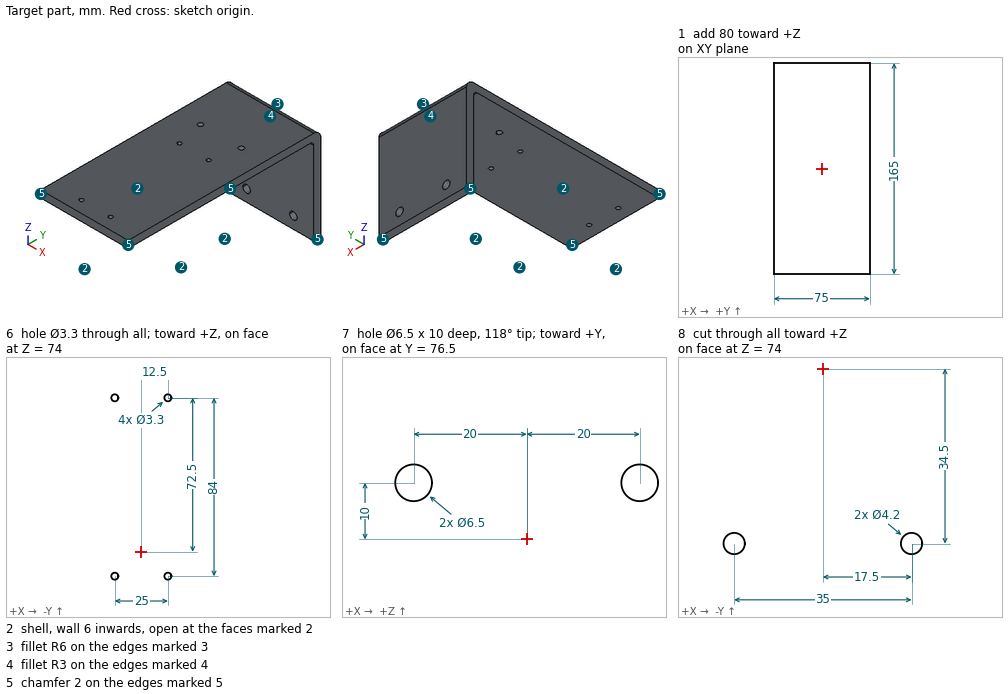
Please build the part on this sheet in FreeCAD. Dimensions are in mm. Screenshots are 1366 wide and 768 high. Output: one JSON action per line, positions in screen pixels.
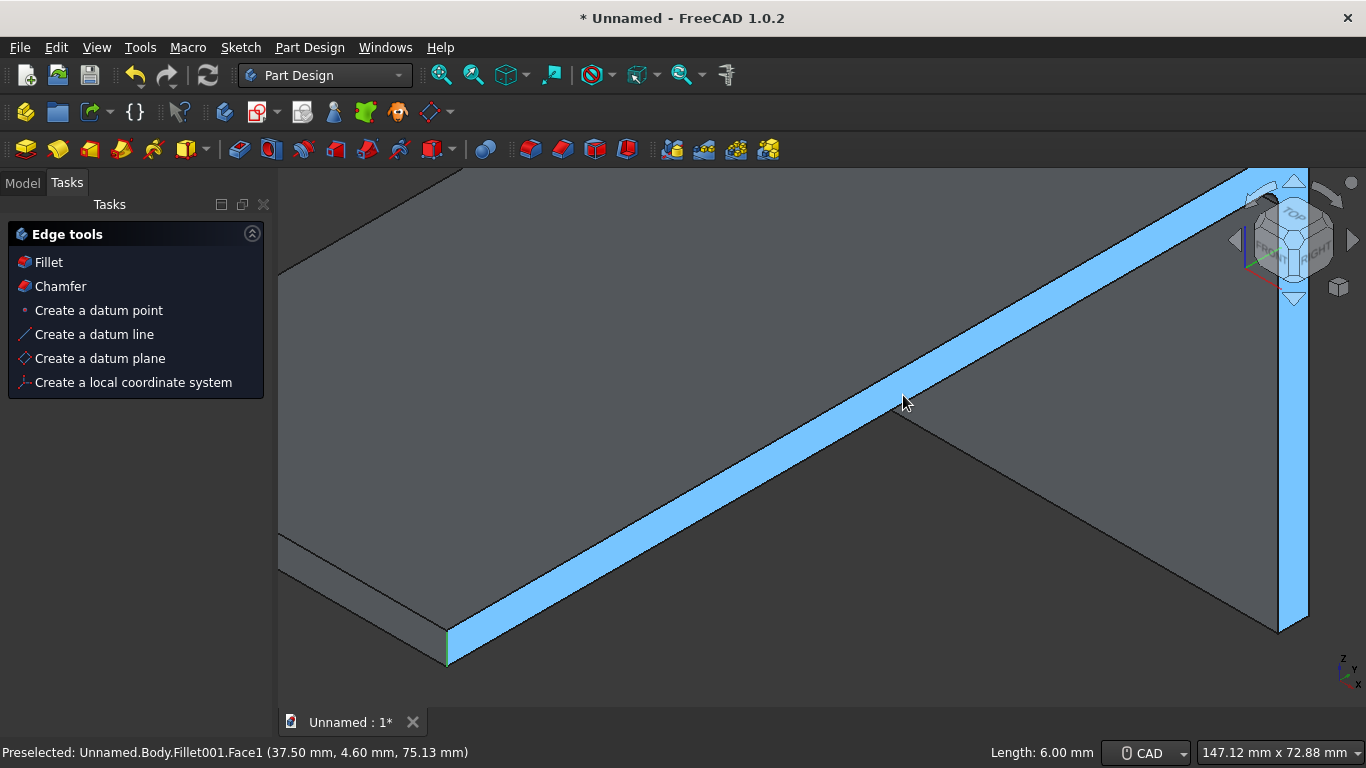
{"action": "left_click", "coordinate": [442, 76]}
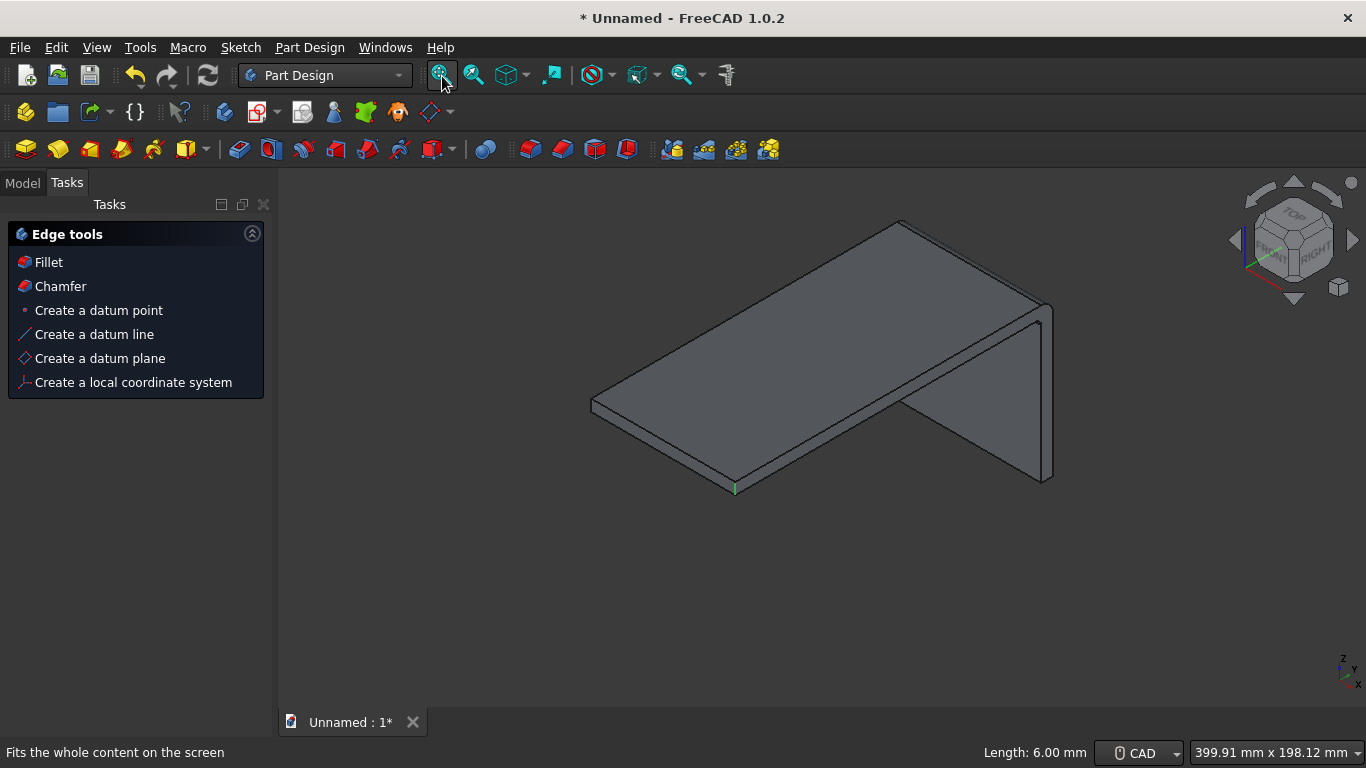
{"action": "key", "text": "1"}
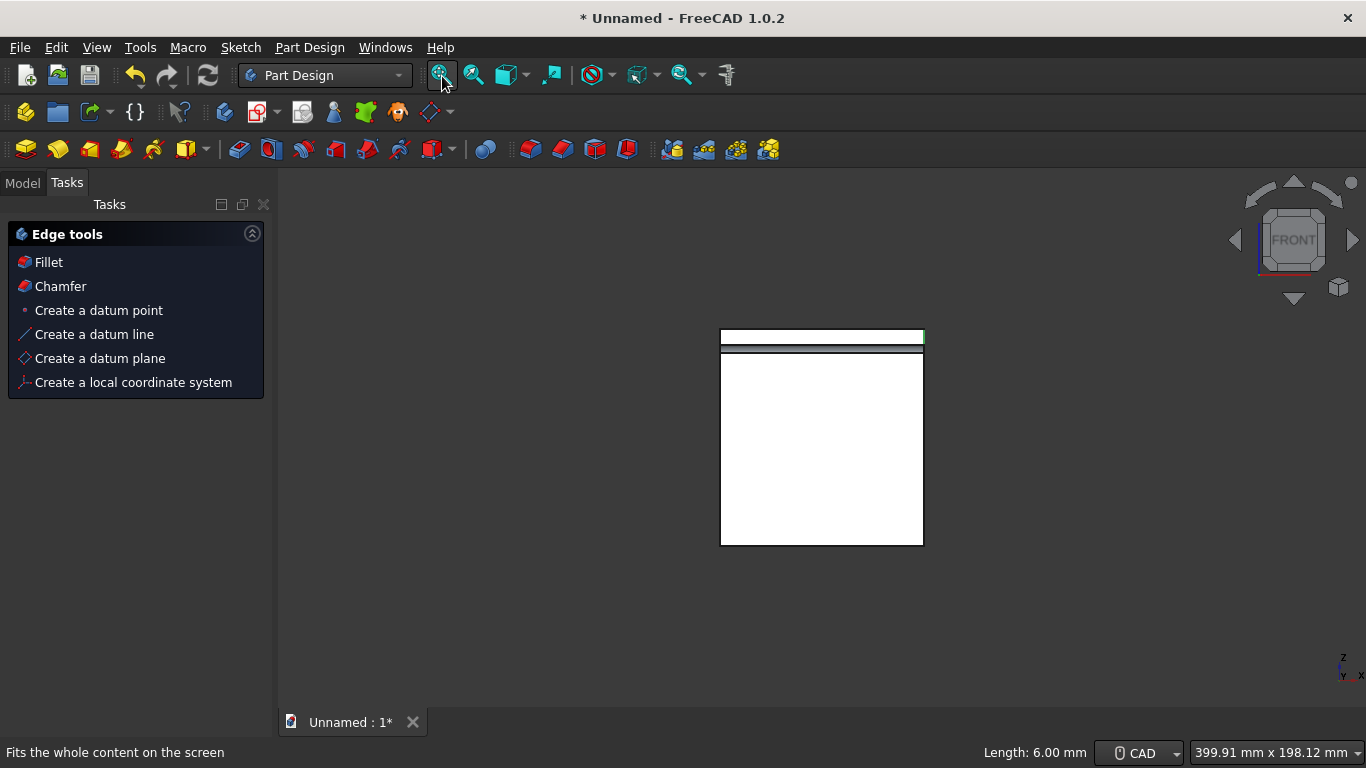
{"action": "left_click", "coordinate": [442, 76]}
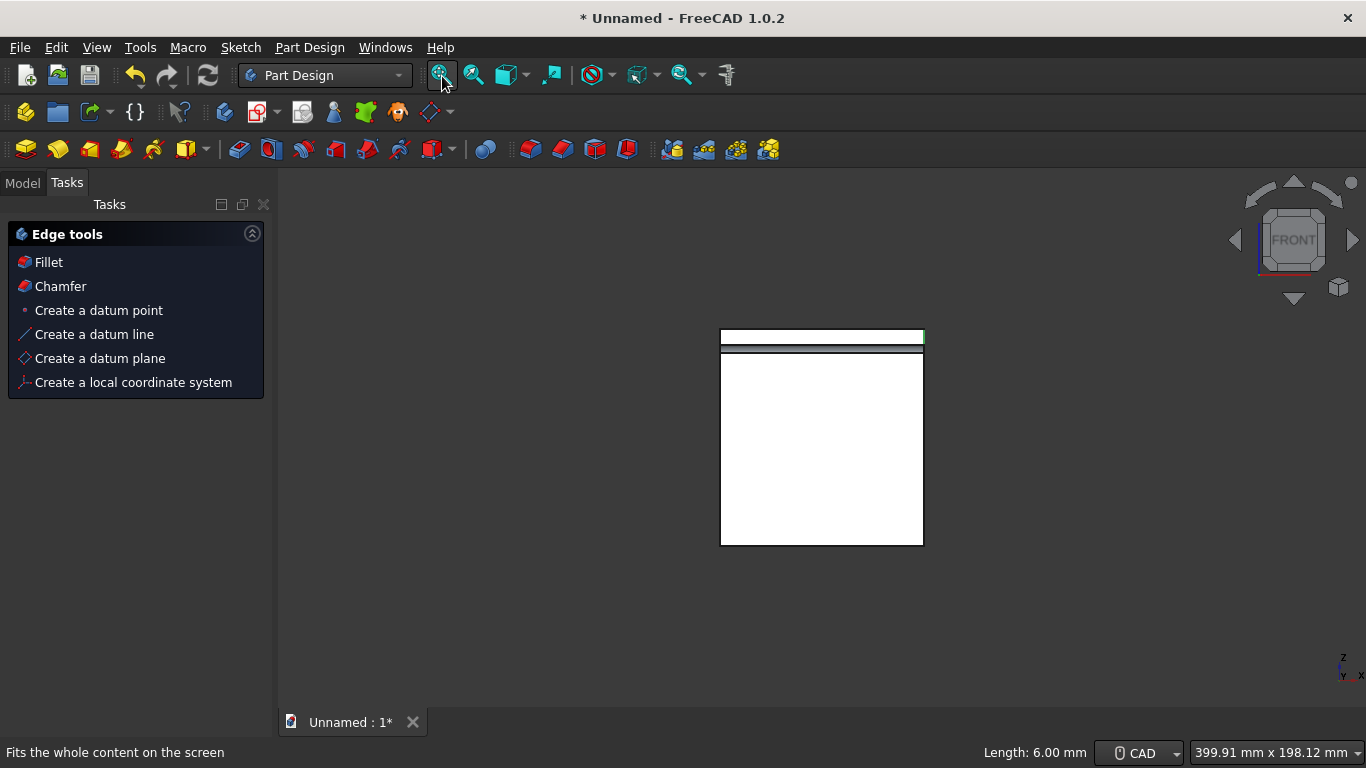
{"action": "left_click", "coordinate": [720, 336], "text": "ctrl"}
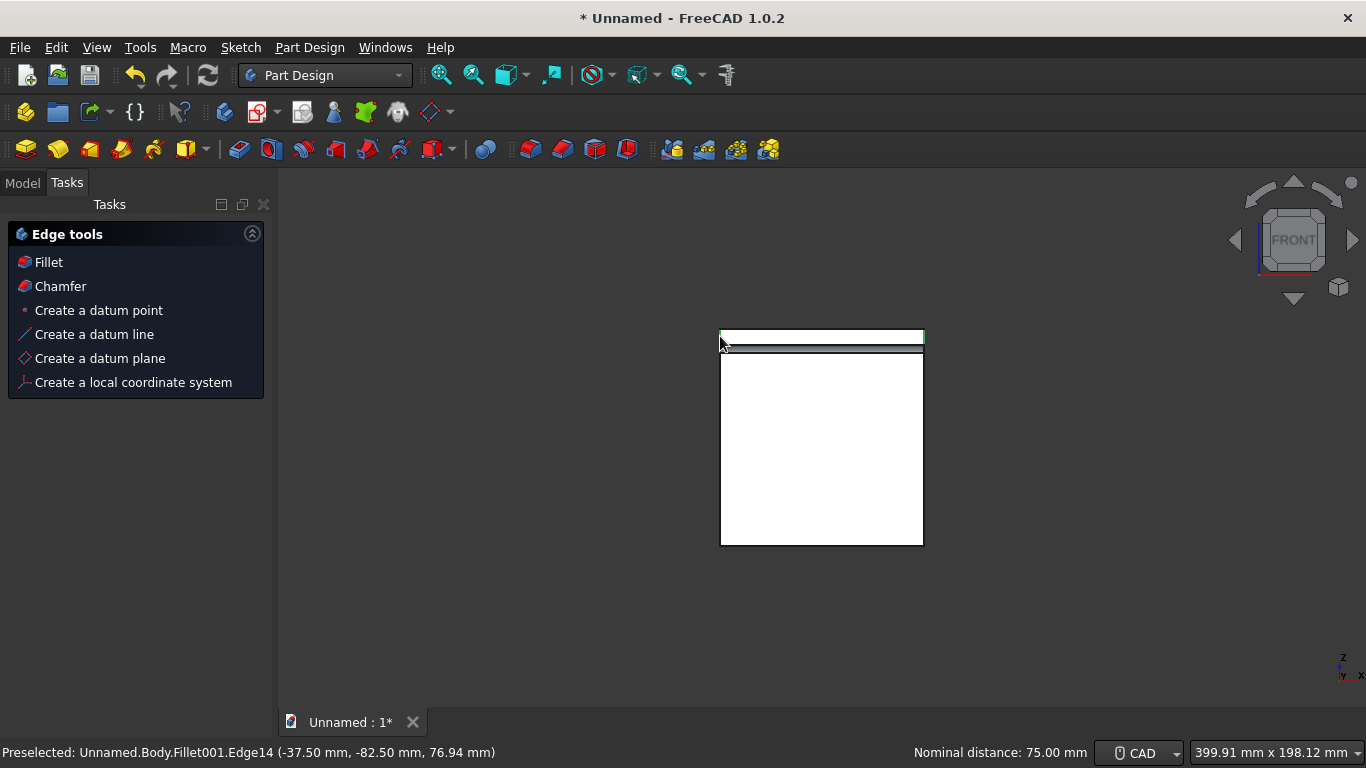
{"action": "scroll", "coordinate": [720, 545], "scroll_direction": "up", "scroll_amount": 5}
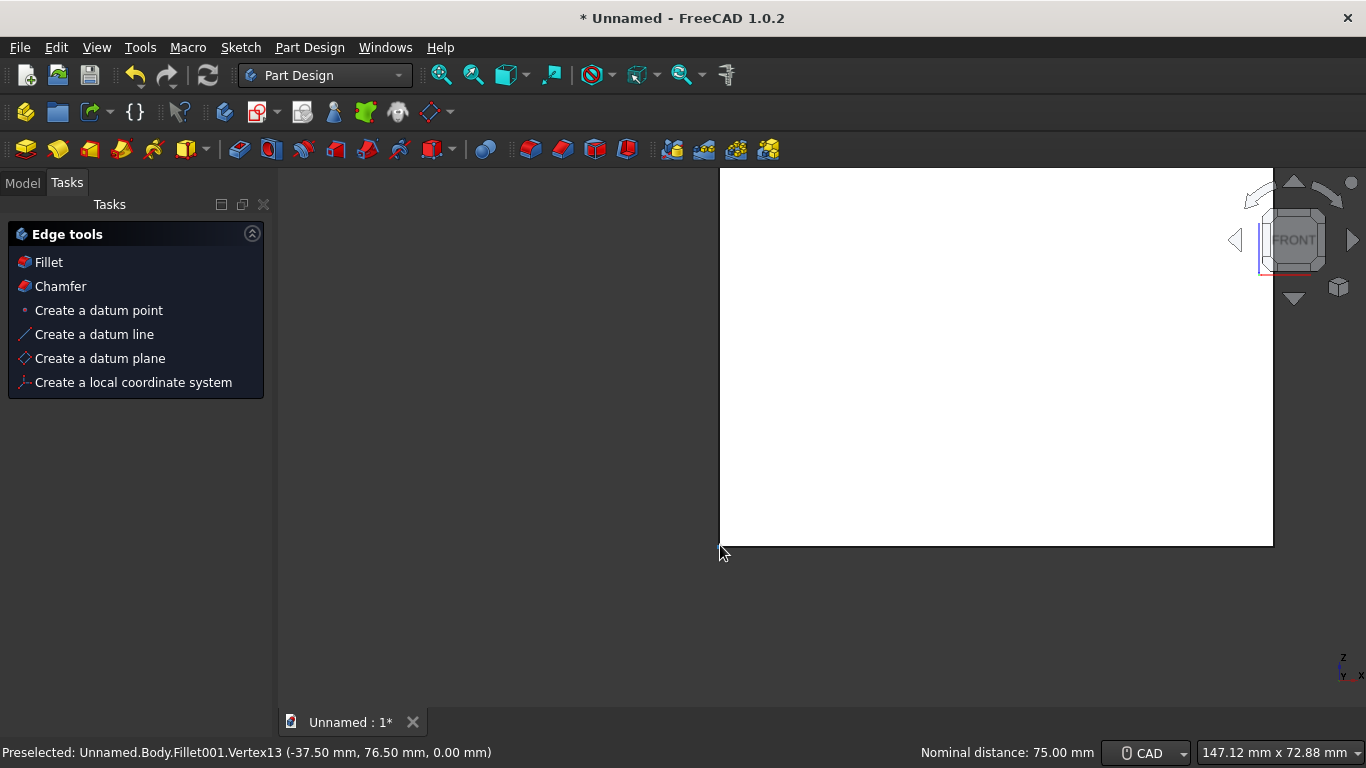
{"action": "left_click", "coordinate": [442, 76]}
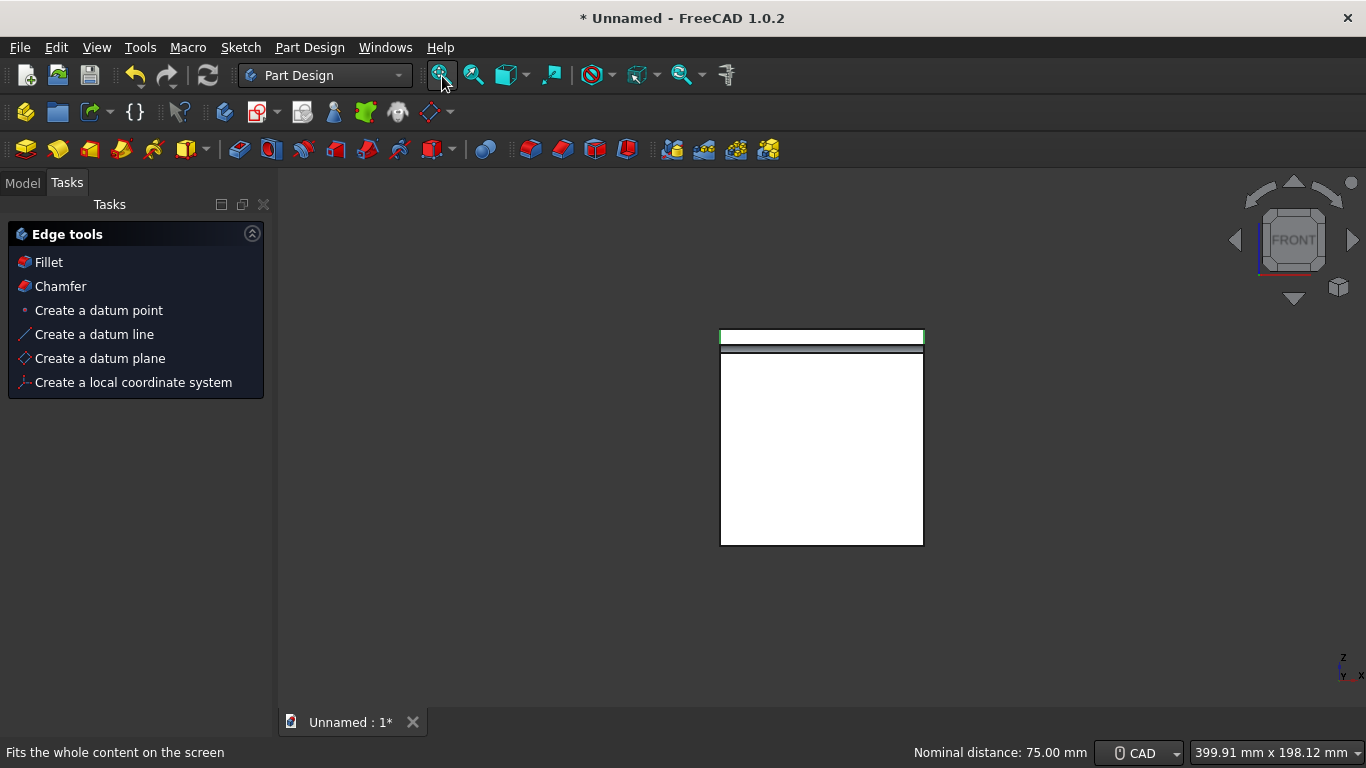
{"action": "key", "text": "3"}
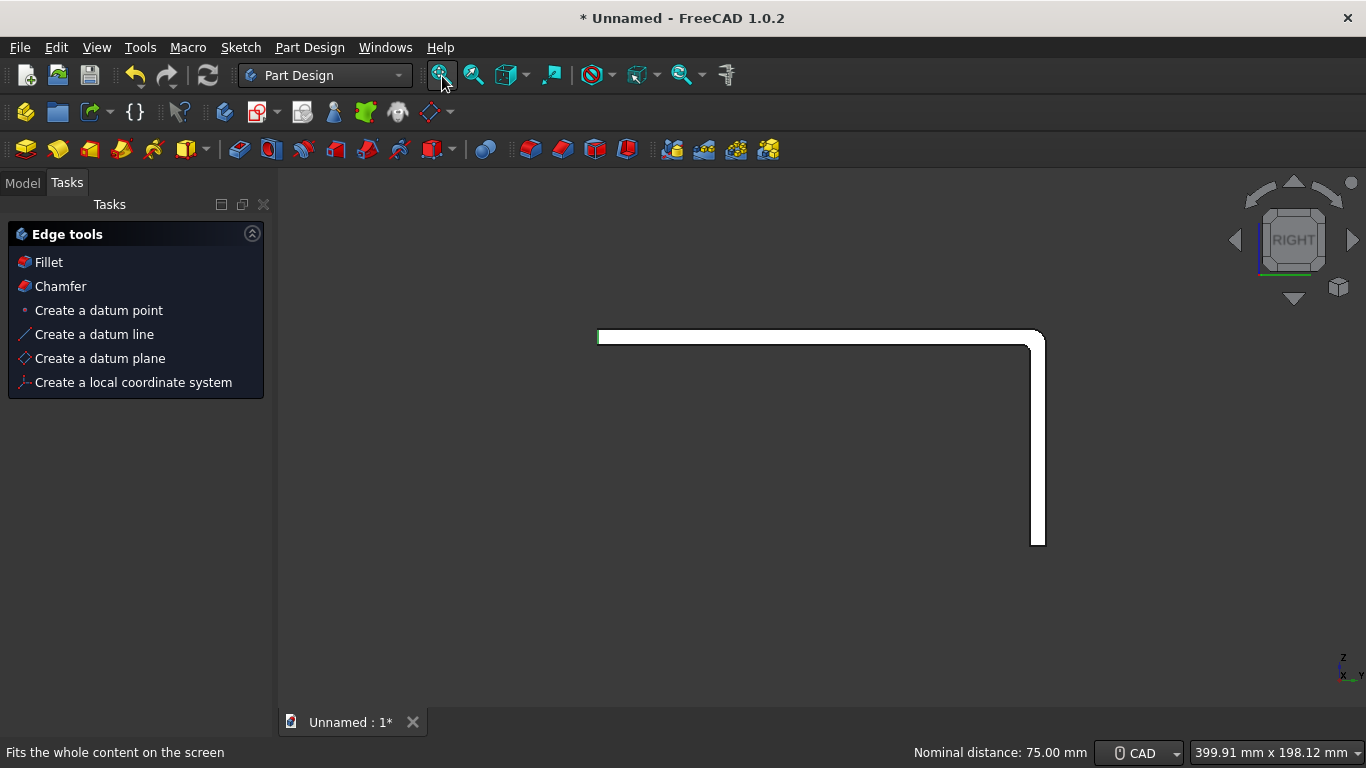
{"action": "left_click", "coordinate": [442, 76]}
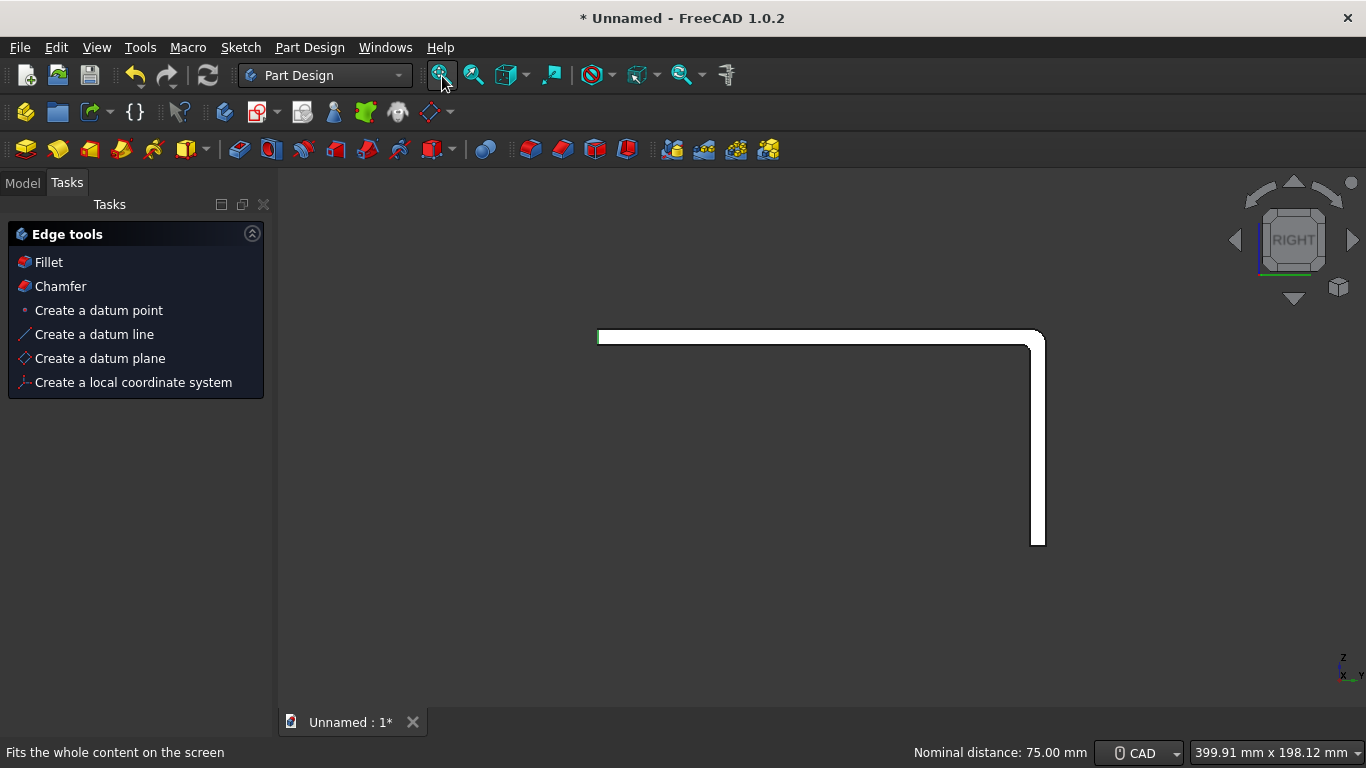
{"action": "left_click", "coordinate": [1038, 545], "text": "ctrl"}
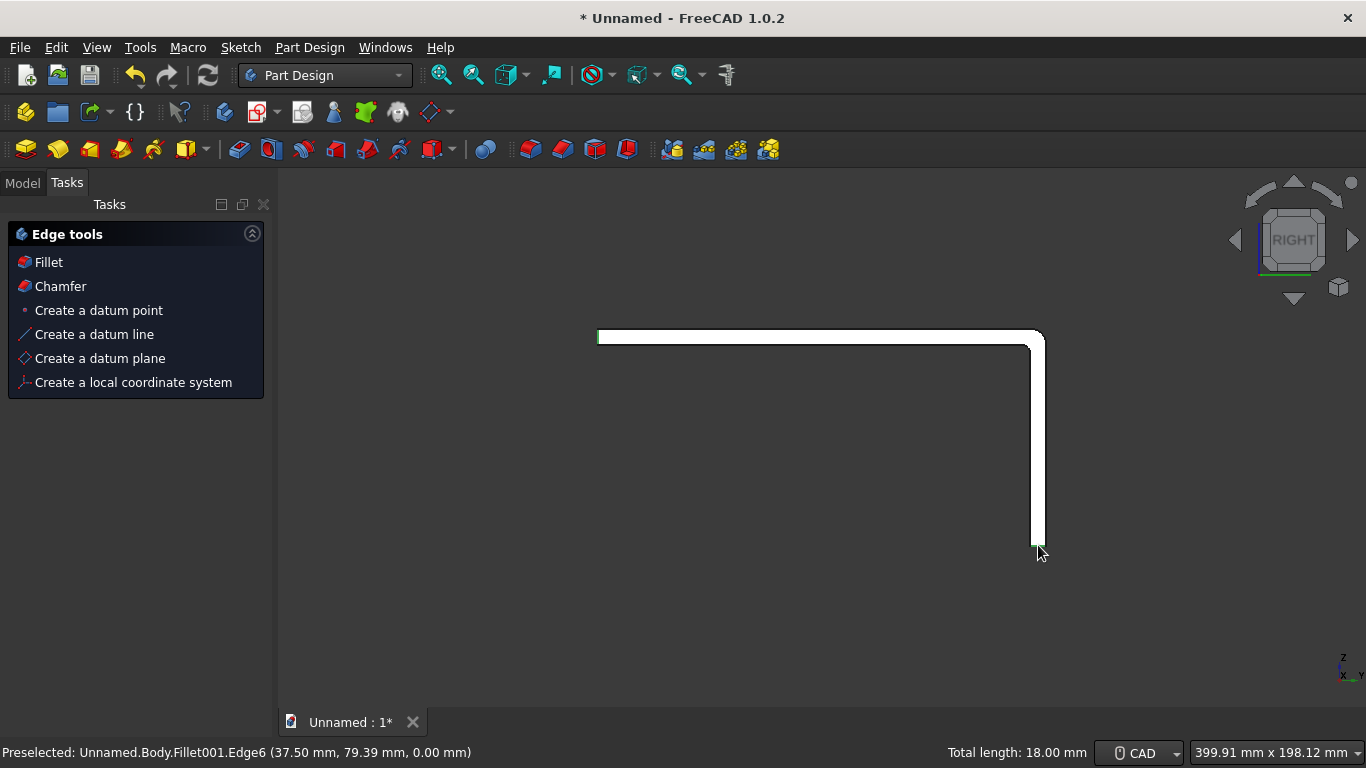
{"action": "scroll", "coordinate": [1038, 545], "scroll_direction": "up", "scroll_amount": 5}